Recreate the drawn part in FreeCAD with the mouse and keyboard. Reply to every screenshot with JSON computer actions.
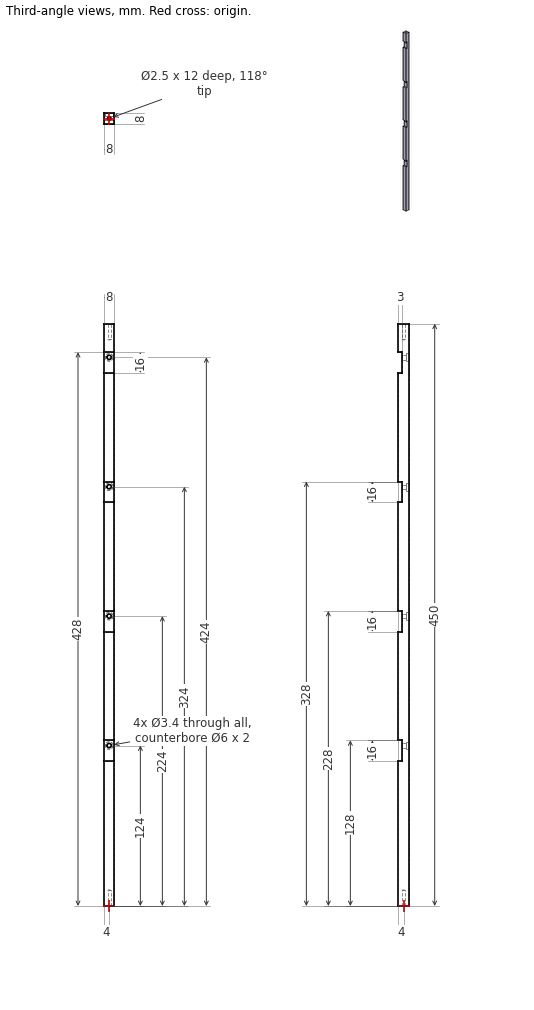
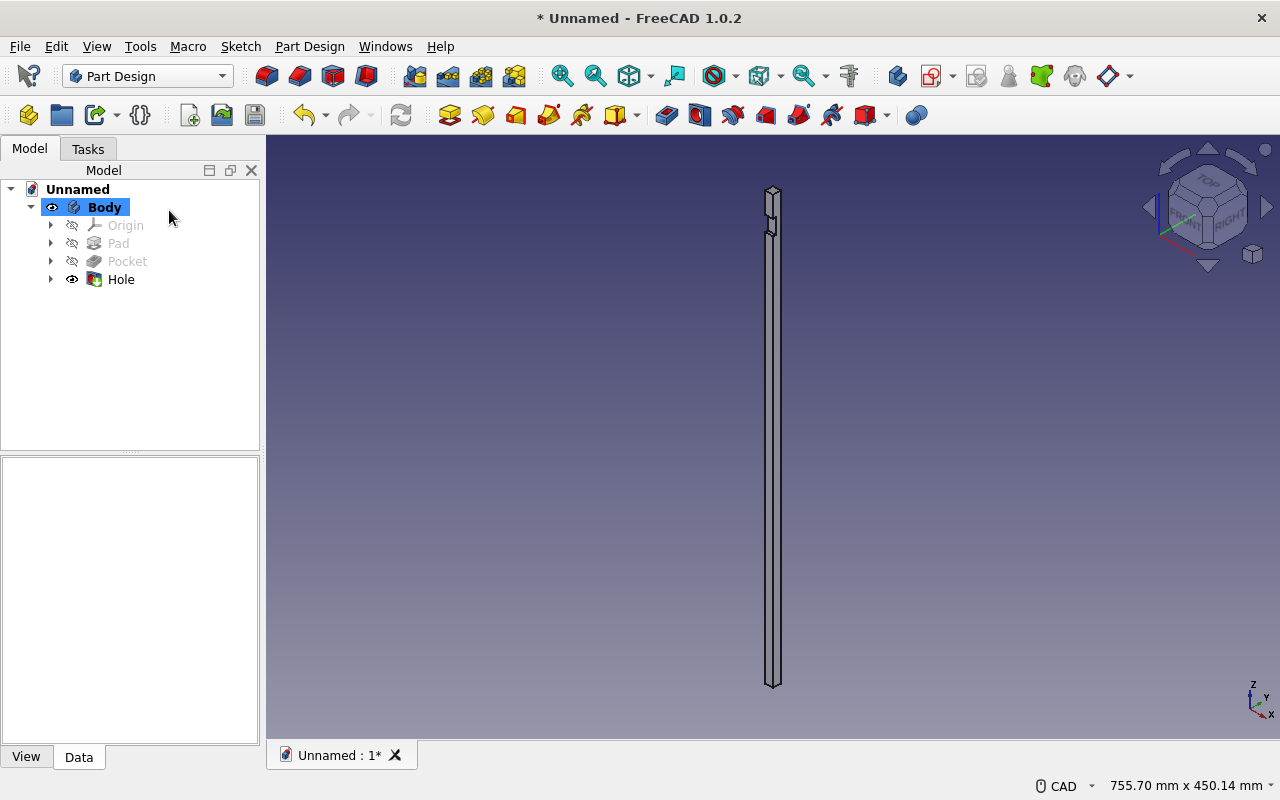
{"action": "scroll", "coordinate": [773, 189], "scroll_direction": "up", "scroll_amount": 5}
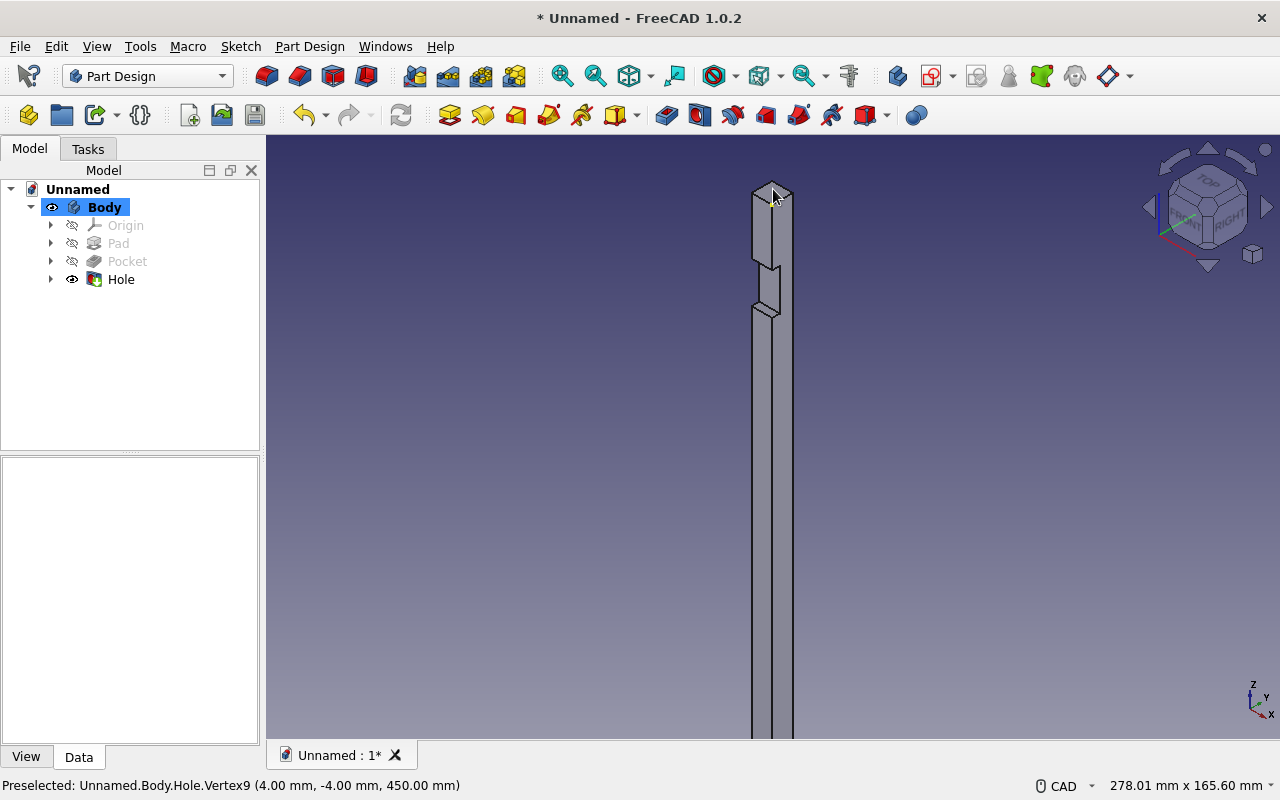
{"action": "left_click", "coordinate": [772, 192]}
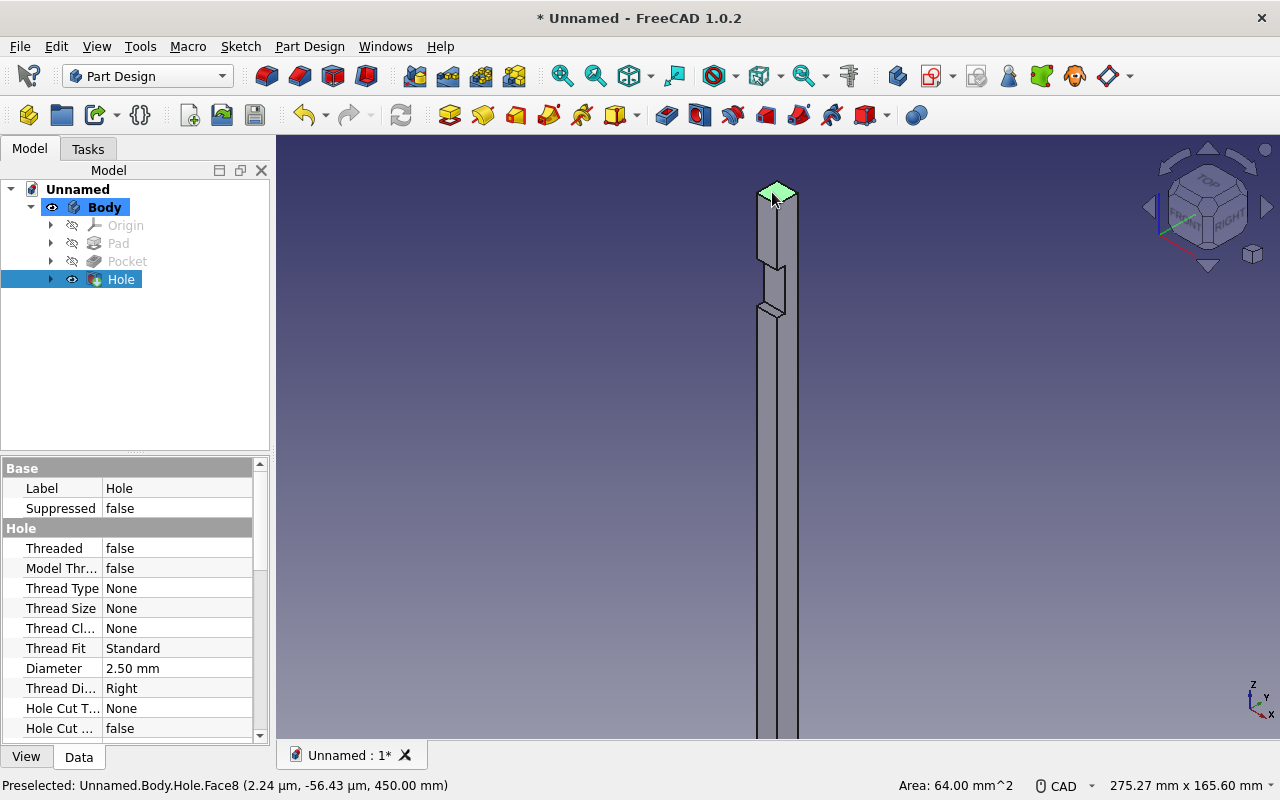
{"action": "left_click", "coordinate": [930, 76]}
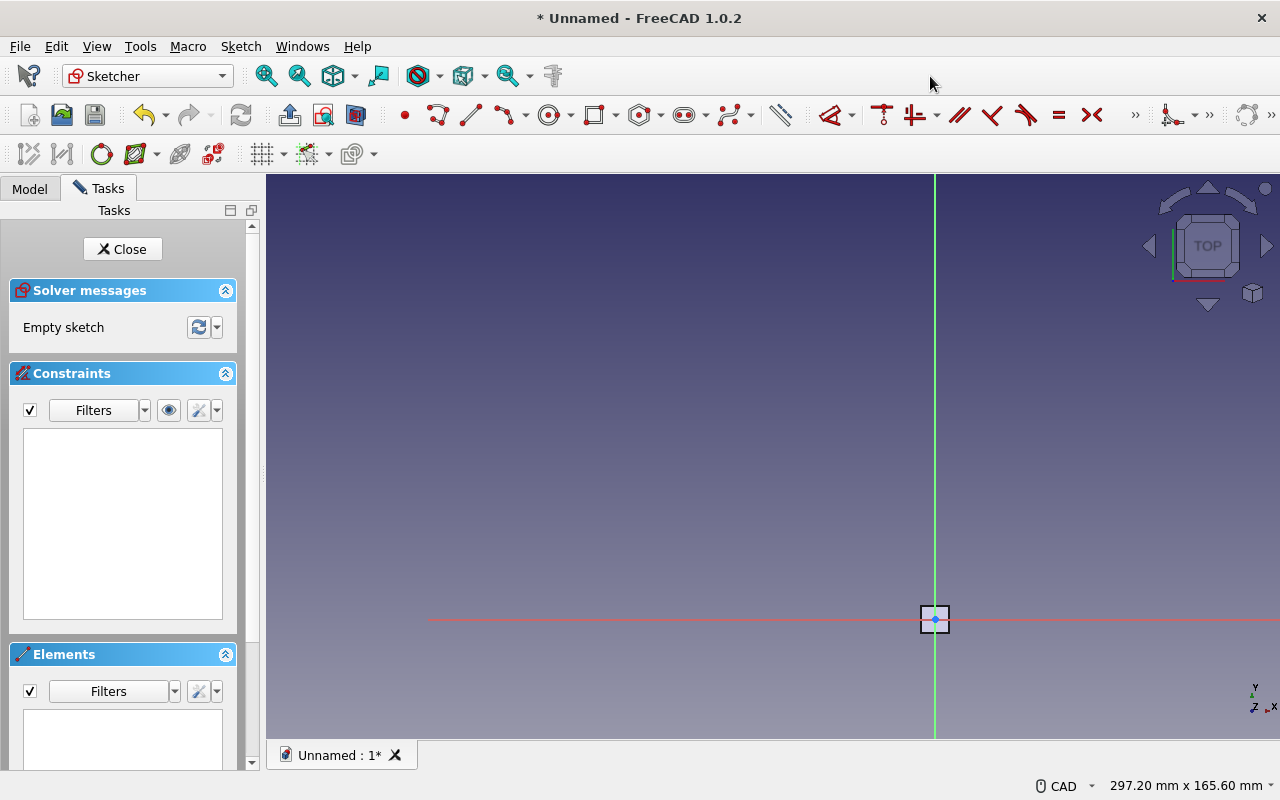
{"action": "scroll", "coordinate": [947, 628], "scroll_direction": "up", "scroll_amount": 15}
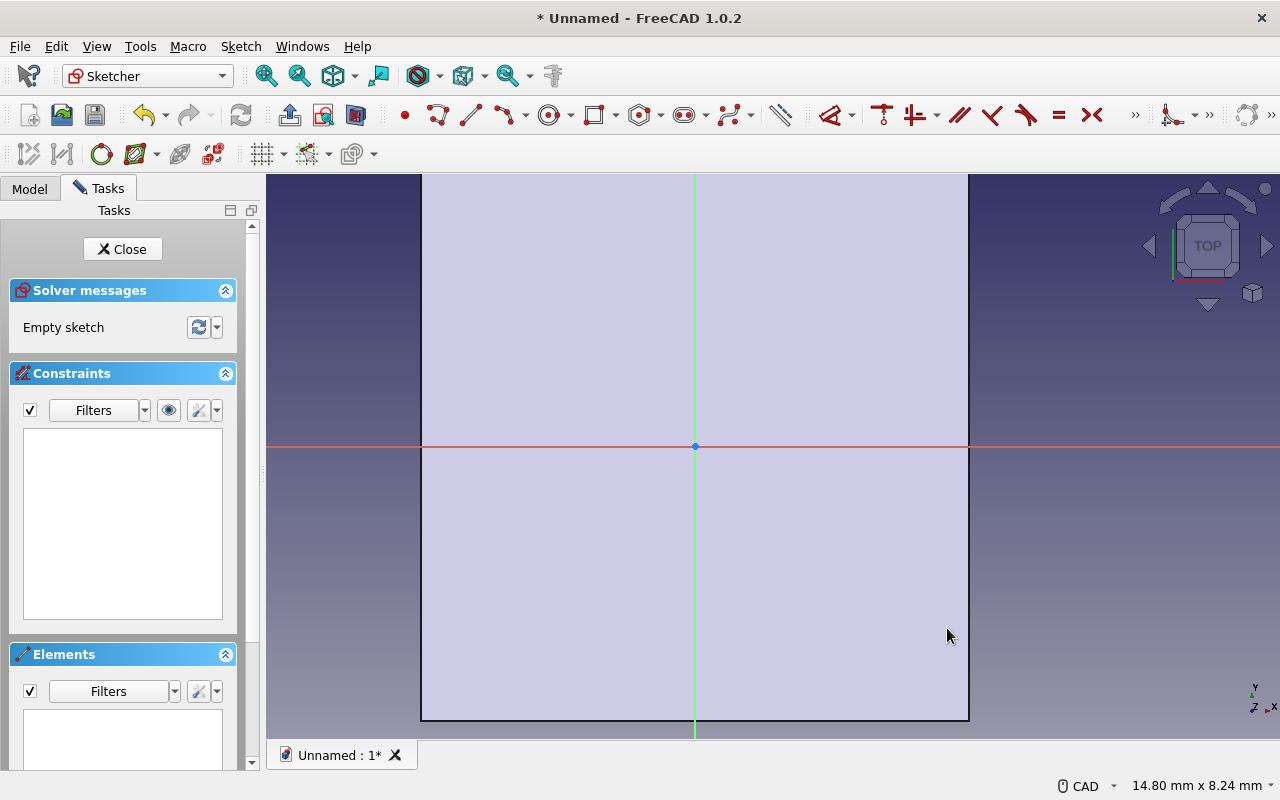
{"action": "scroll", "coordinate": [688, 439], "scroll_direction": "up", "scroll_amount": 4}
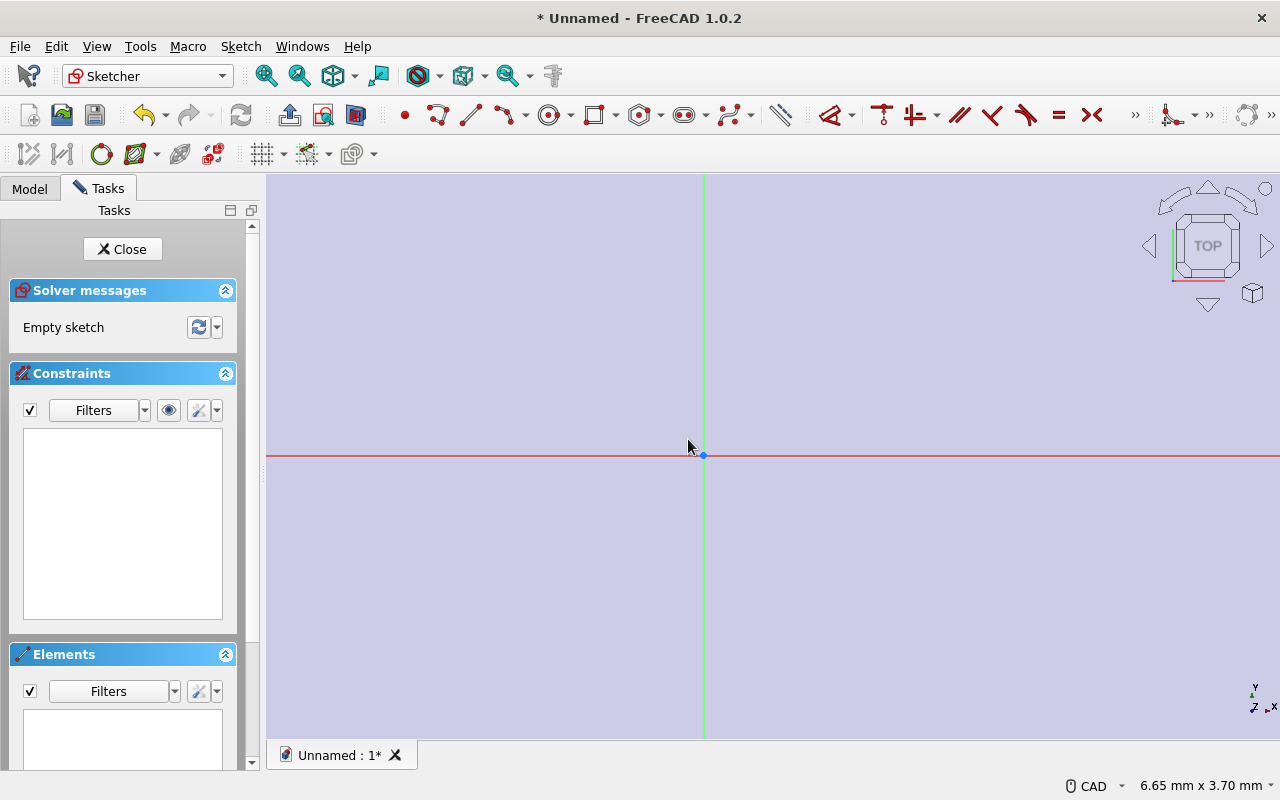
{"action": "left_click", "coordinate": [548, 116]}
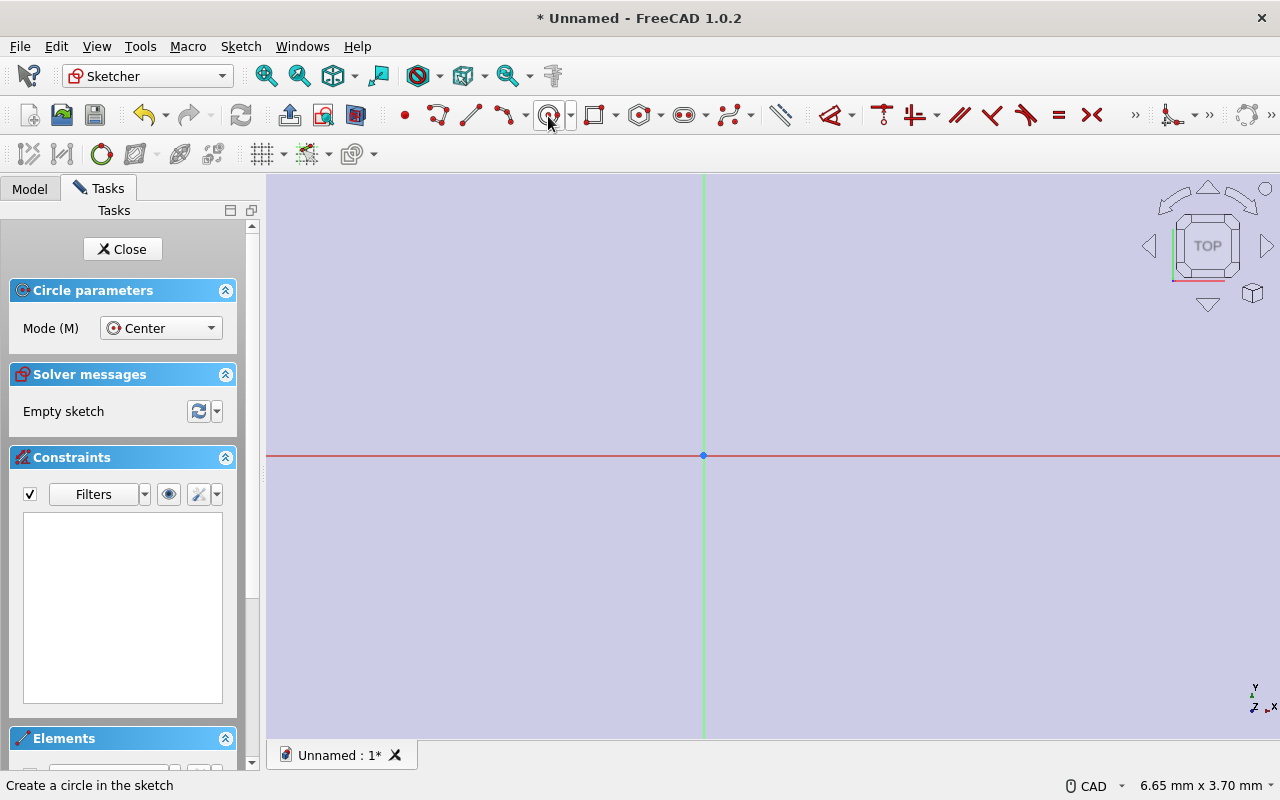
{"action": "left_click", "coordinate": [704, 456]}
{"action": "mouse_move", "coordinate": [839, 321]}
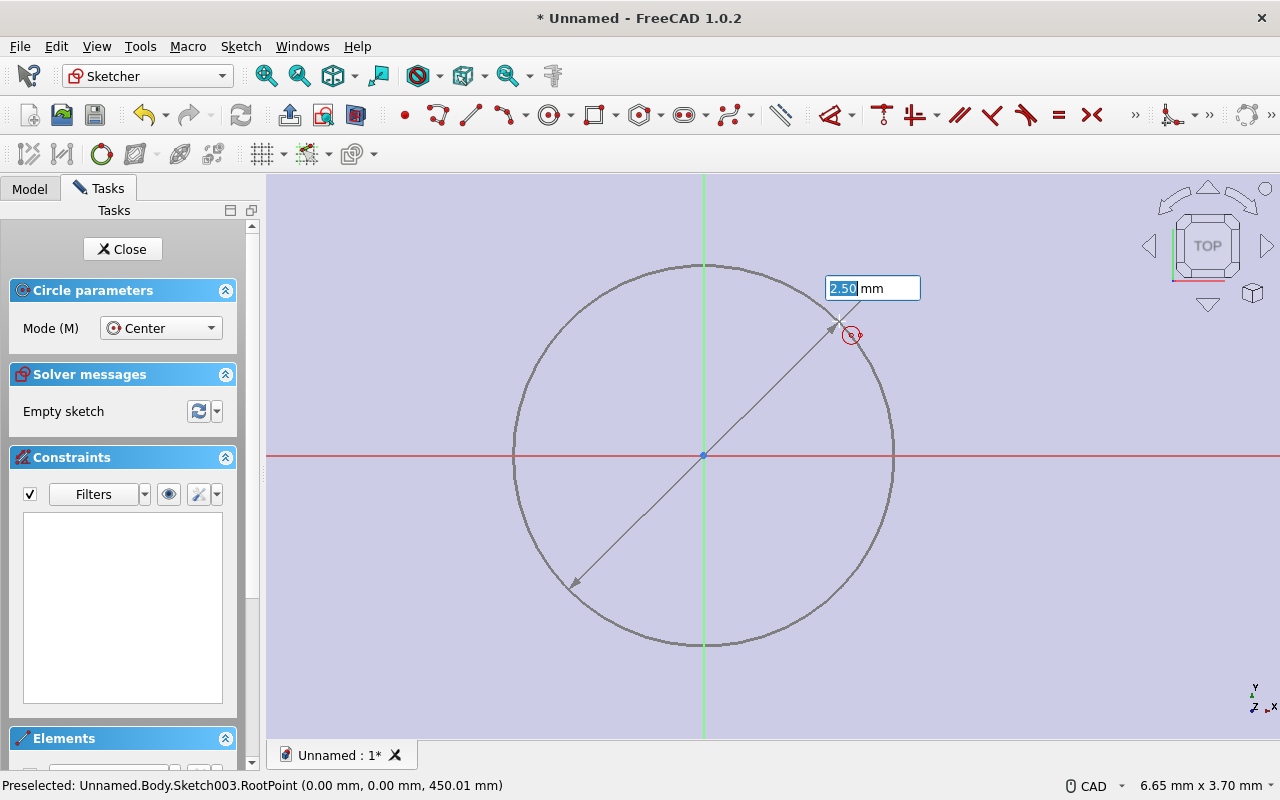
{"action": "type", "text": "2.5"}
{"action": "key", "text": "Return"}
{"action": "key", "text": "Escape"}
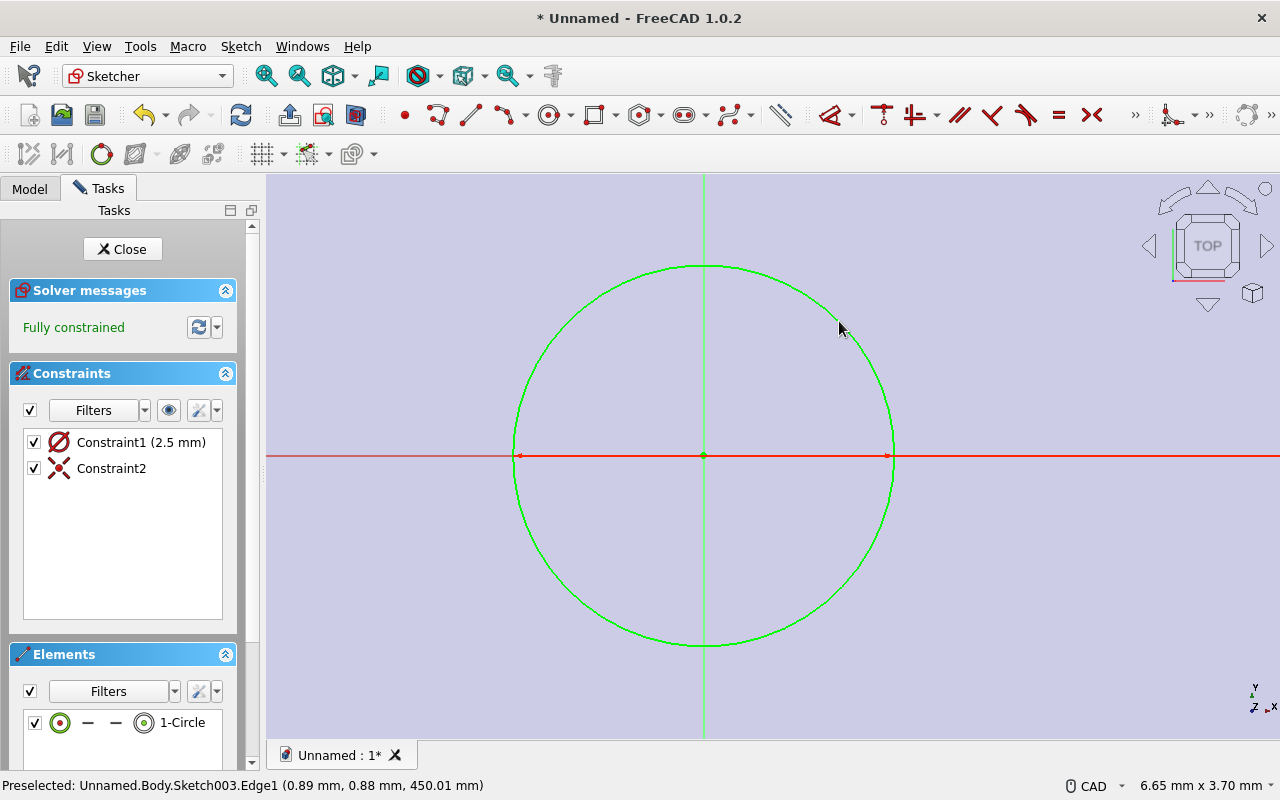
{"action": "left_click", "coordinate": [123, 249]}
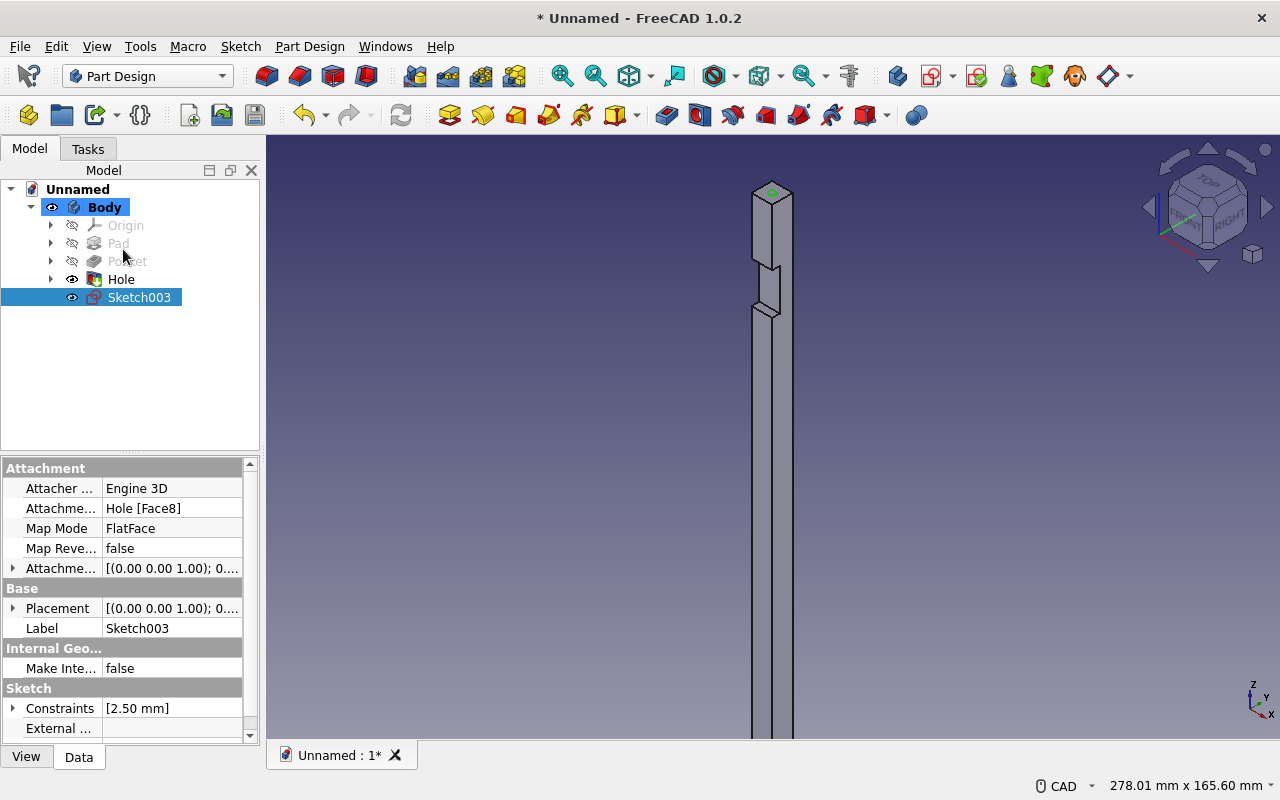
{"action": "left_click", "coordinate": [700, 116]}